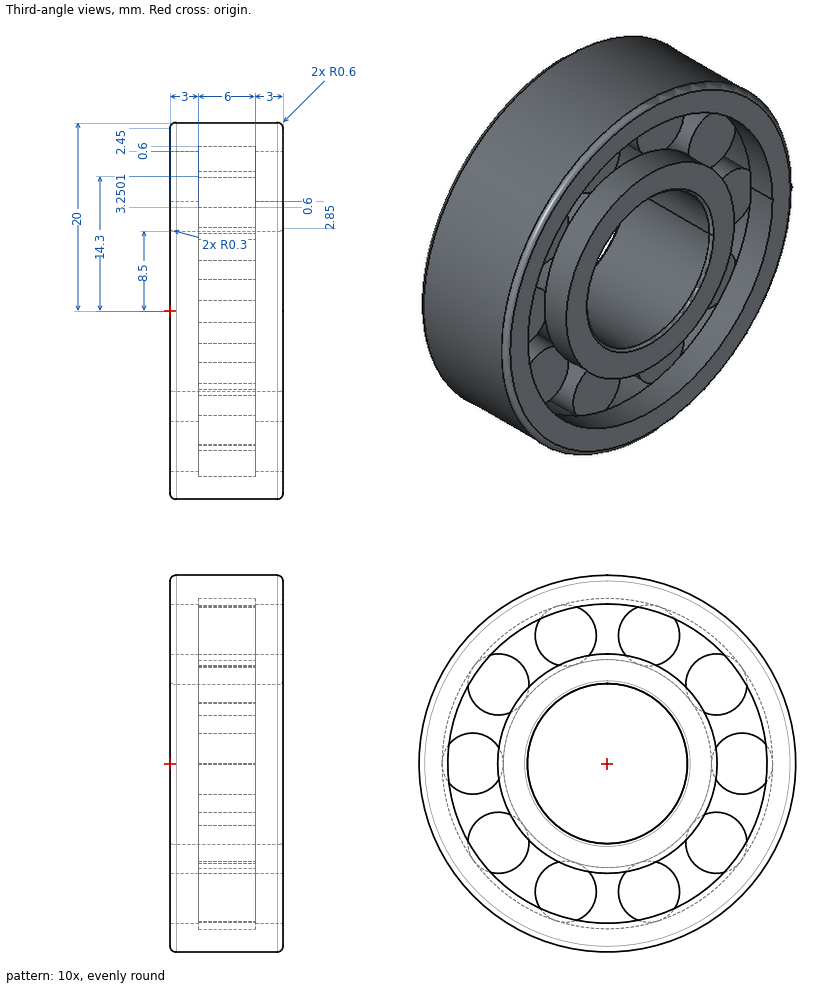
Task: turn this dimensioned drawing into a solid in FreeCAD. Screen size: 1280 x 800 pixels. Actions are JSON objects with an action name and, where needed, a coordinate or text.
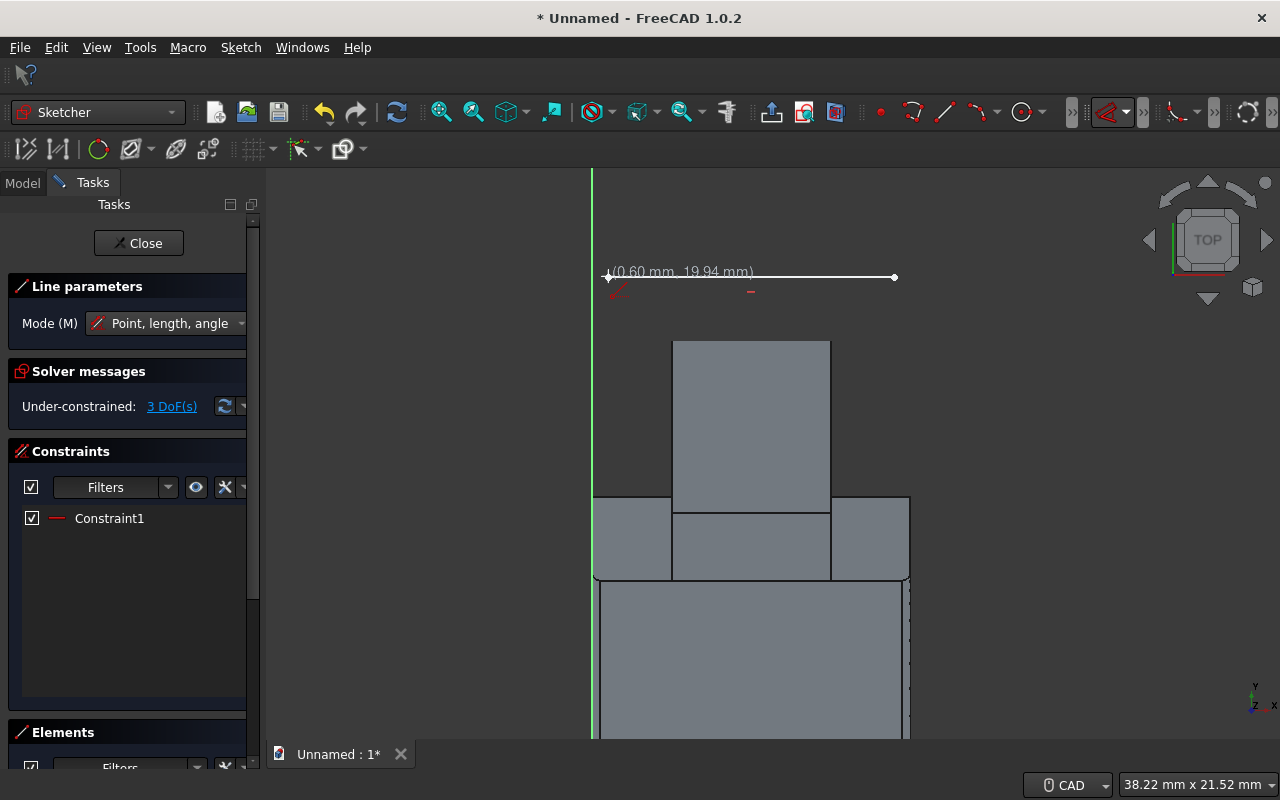
{"action": "left_click", "coordinate": [914, 112]}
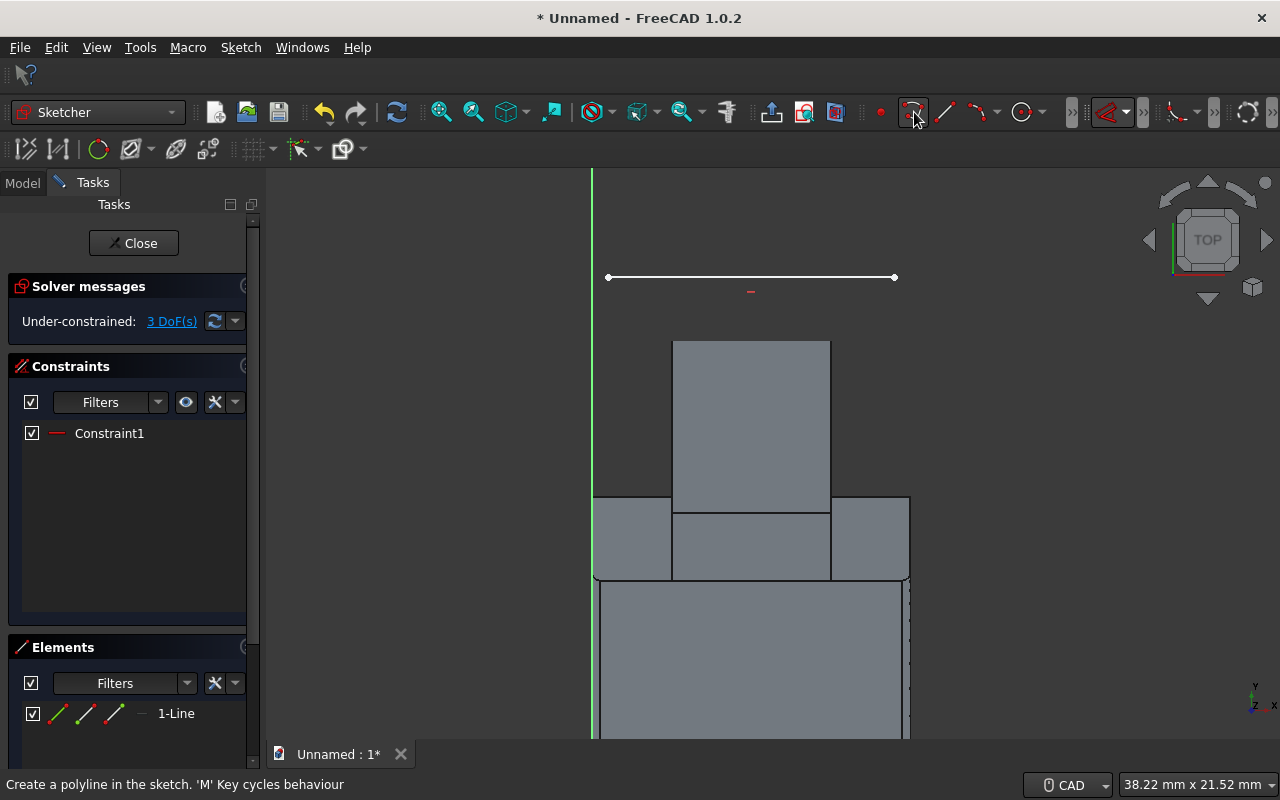
{"action": "left_click", "coordinate": [592, 291]}
{"action": "left_click", "coordinate": [601, 356]}
{"action": "left_click", "coordinate": [672, 356]}
{"action": "left_click", "coordinate": [672, 340]}
{"action": "left_click", "coordinate": [831, 340]}
{"action": "left_click", "coordinate": [831, 356]}
{"action": "left_click", "coordinate": [910, 356]}
{"action": "left_click", "coordinate": [910, 291]}
{"action": "right_click", "coordinate": [910, 291]}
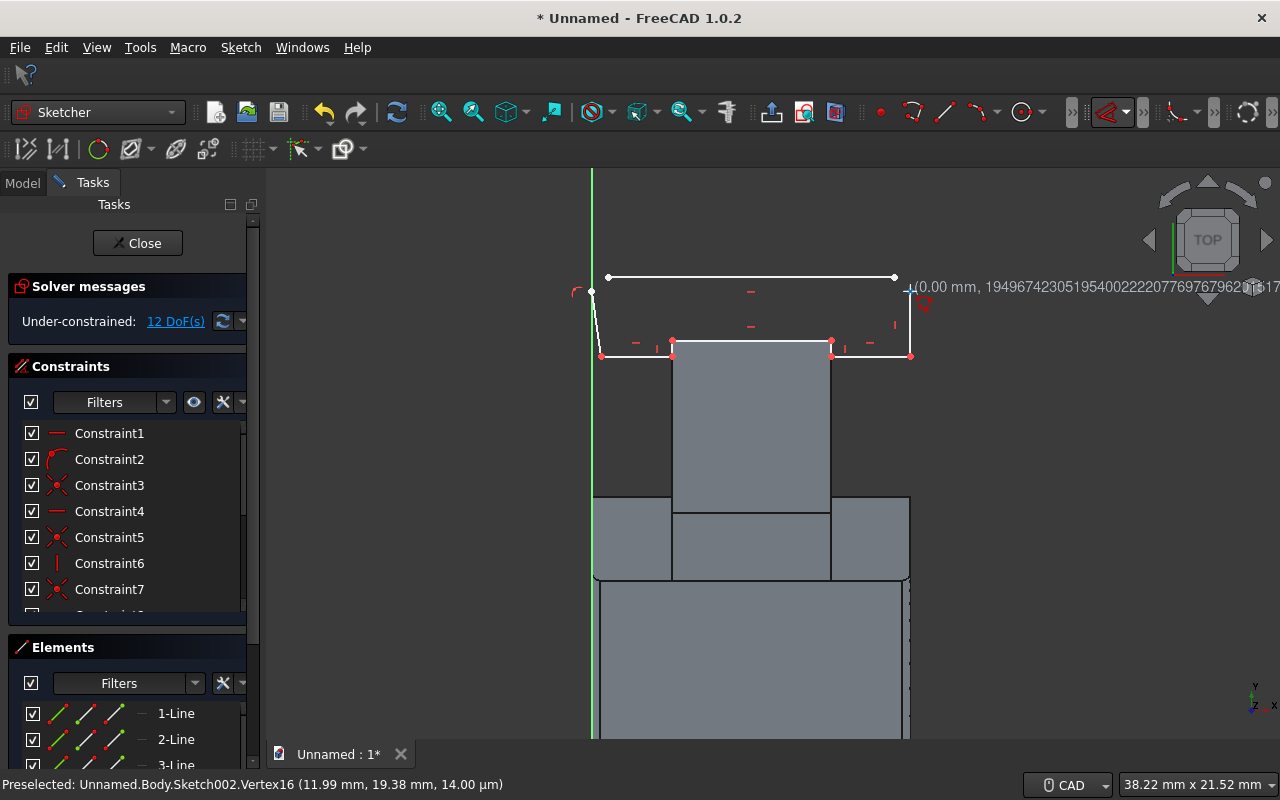
{"action": "left_click", "coordinate": [978, 112]}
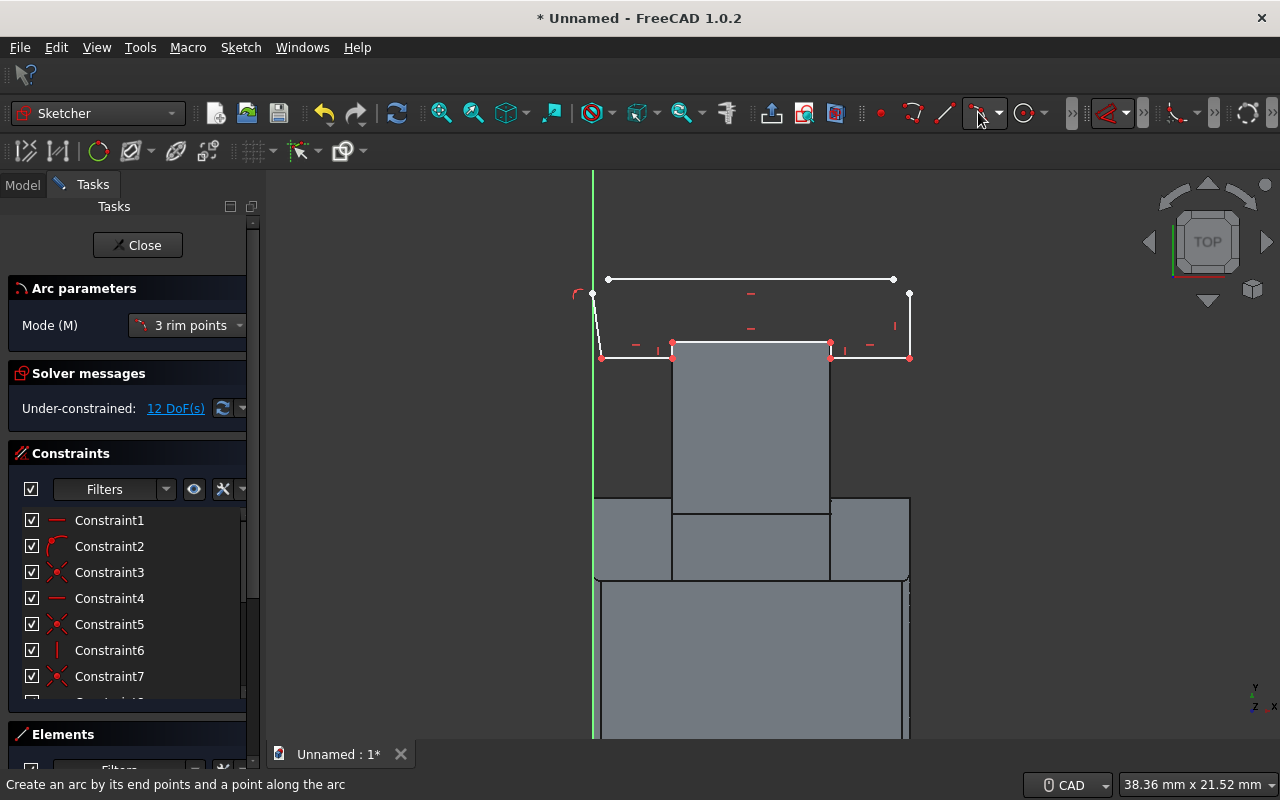
{"action": "left_click", "coordinate": [609, 279]}
{"action": "left_click", "coordinate": [593, 294]}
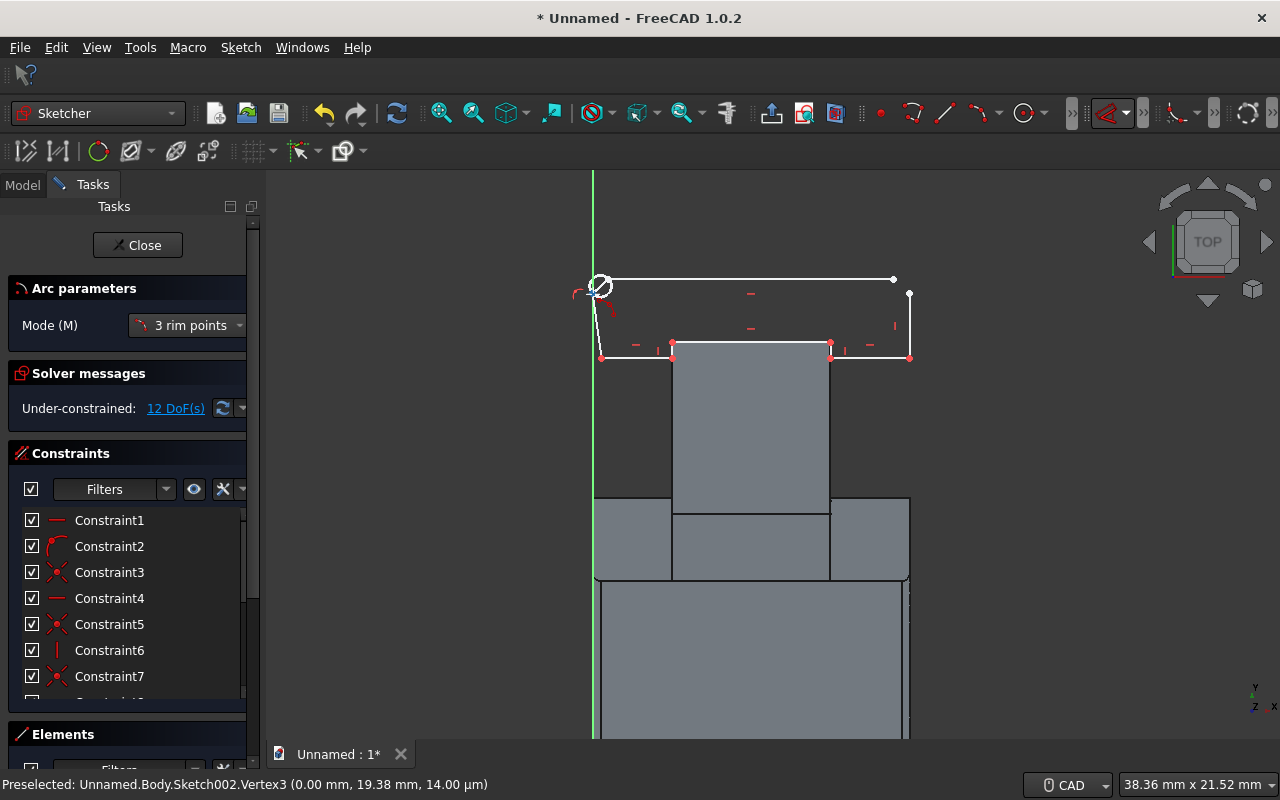
{"action": "scroll", "coordinate": [597, 282], "scroll_direction": "up", "scroll_amount": 7}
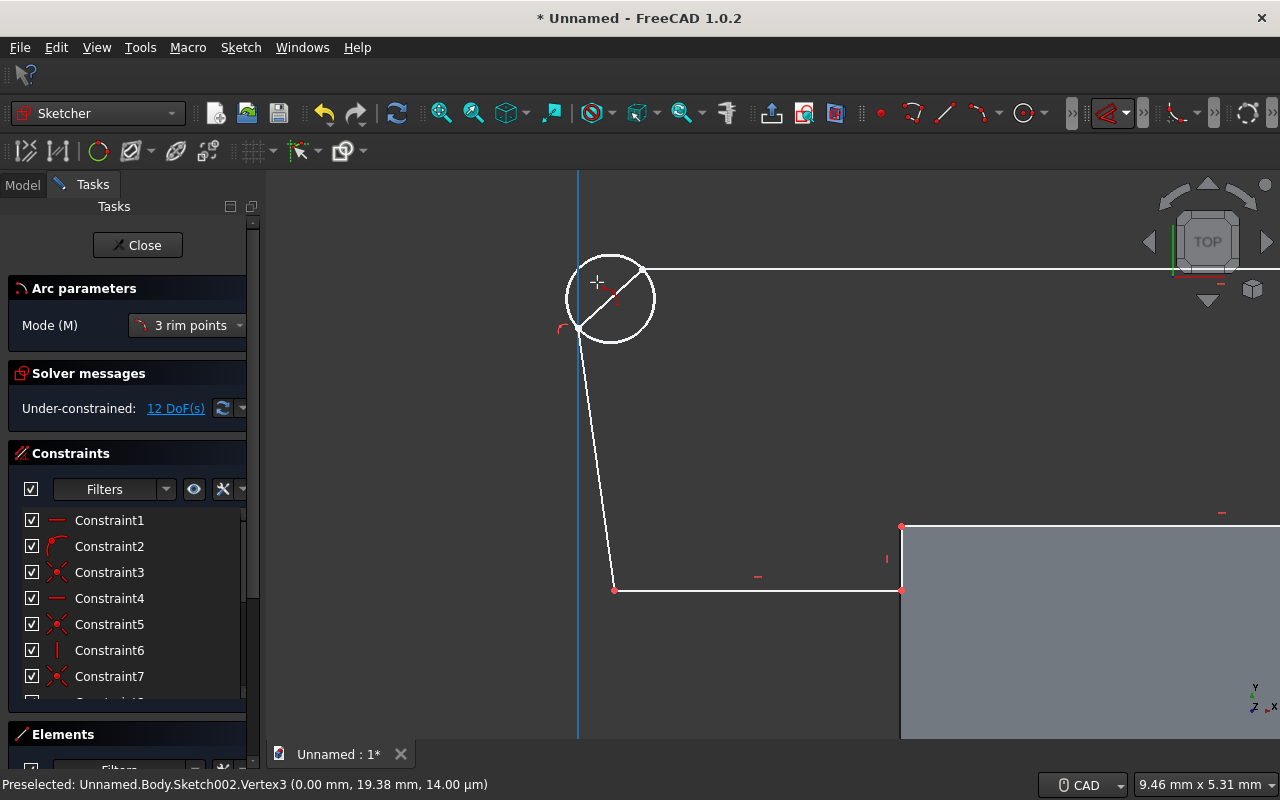
{"action": "left_click", "coordinate": [597, 280]}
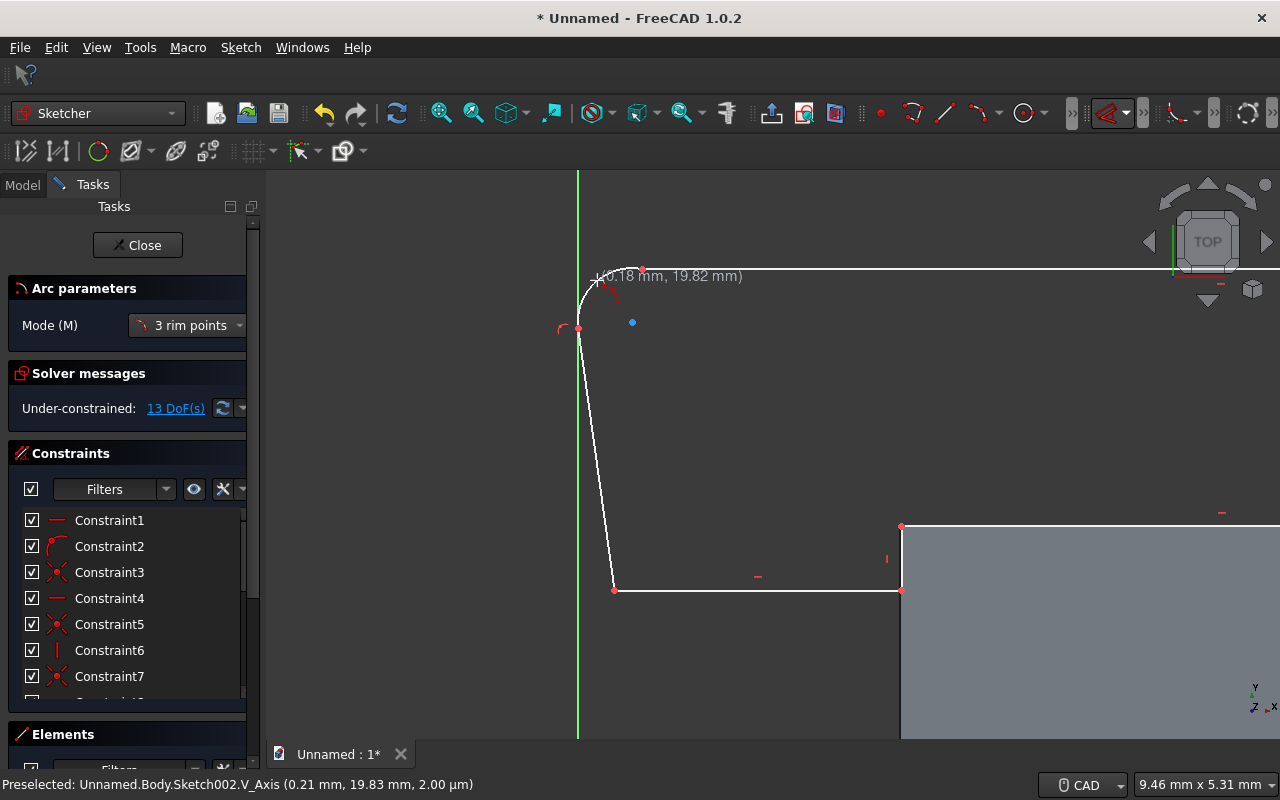
{"action": "scroll", "coordinate": [602, 280], "scroll_direction": "down", "scroll_amount": 9}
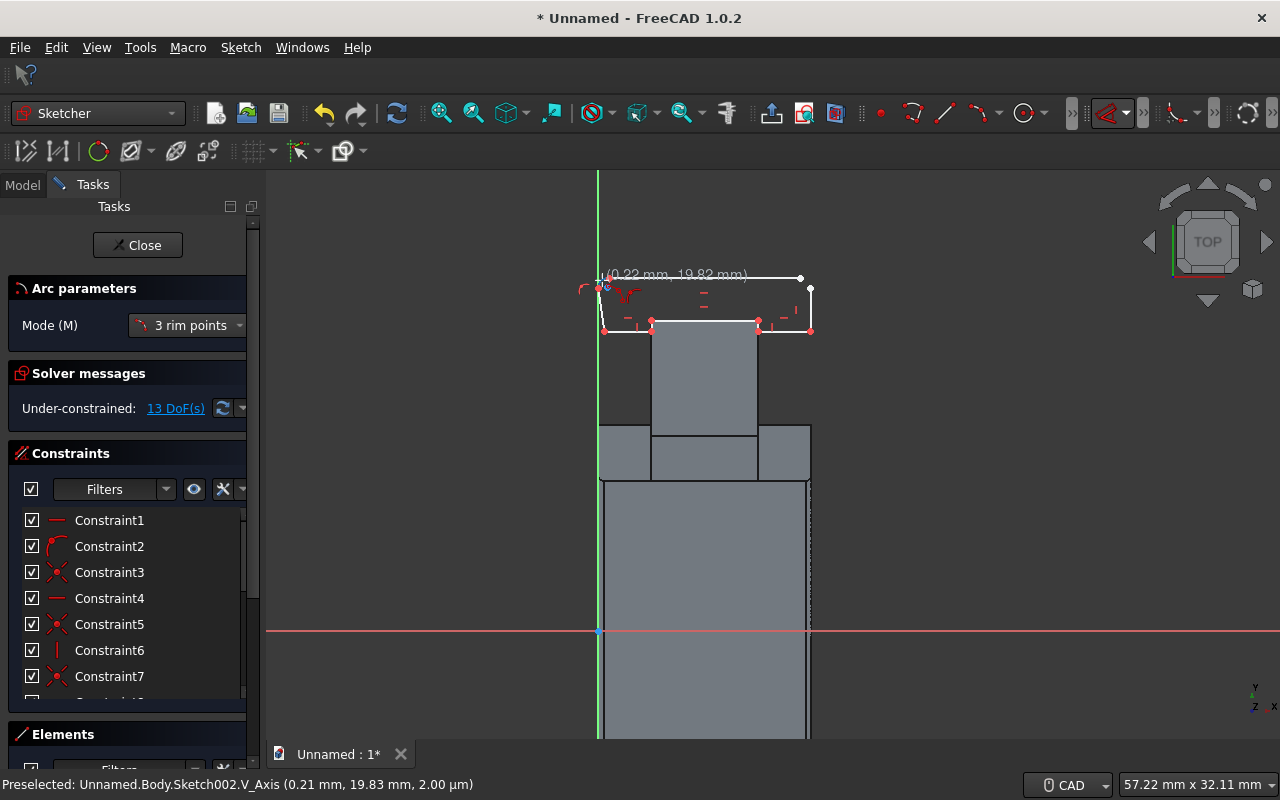
{"action": "left_click", "coordinate": [811, 288]}
{"action": "left_click", "coordinate": [800, 278]}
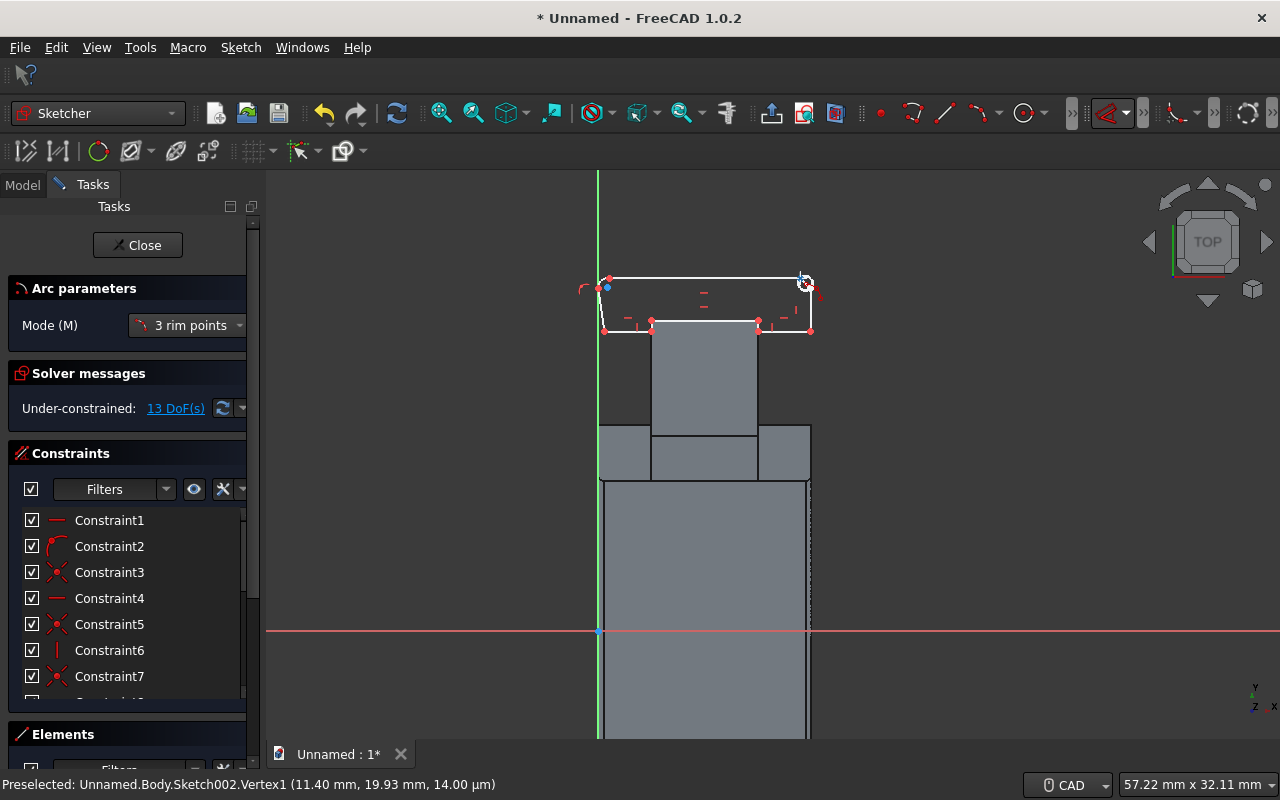
{"action": "scroll", "coordinate": [808, 280], "scroll_direction": "up", "scroll_amount": 9}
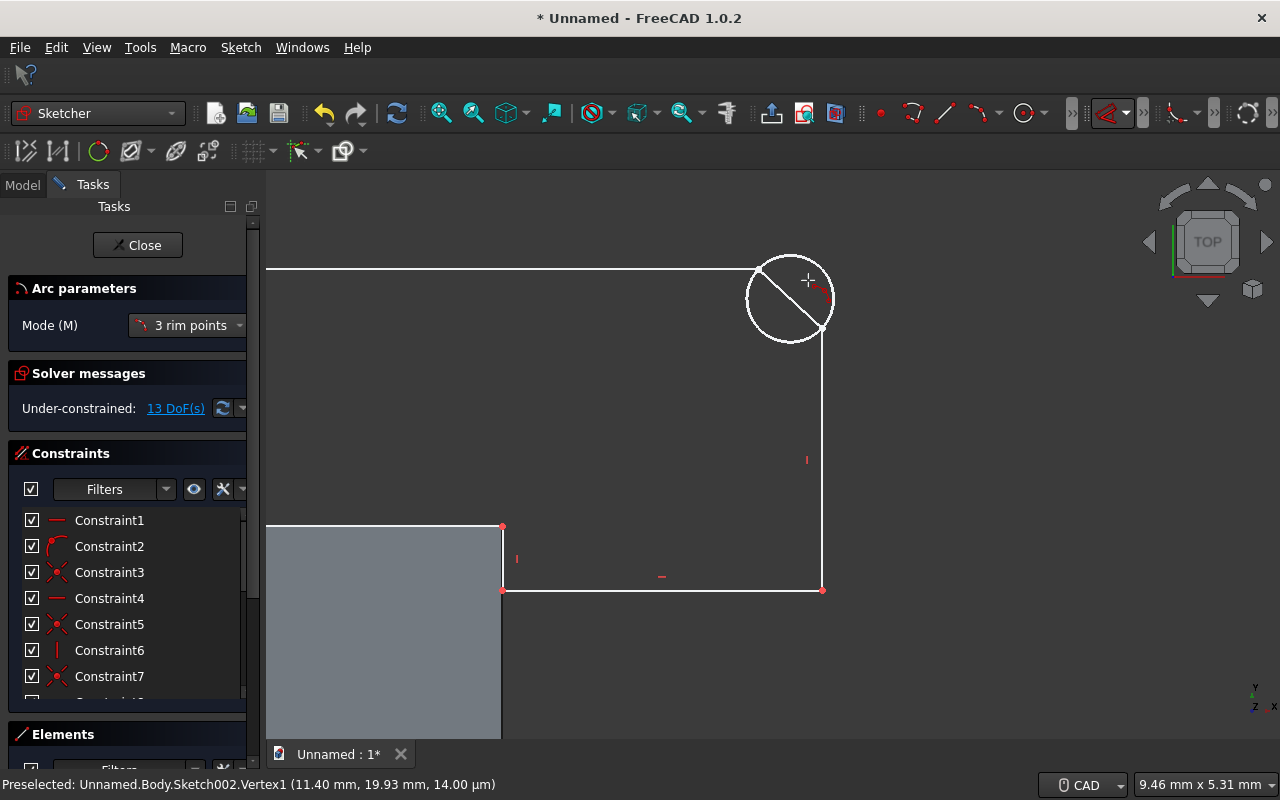
{"action": "left_click", "coordinate": [804, 280]}
{"action": "key", "text": "Escape"}